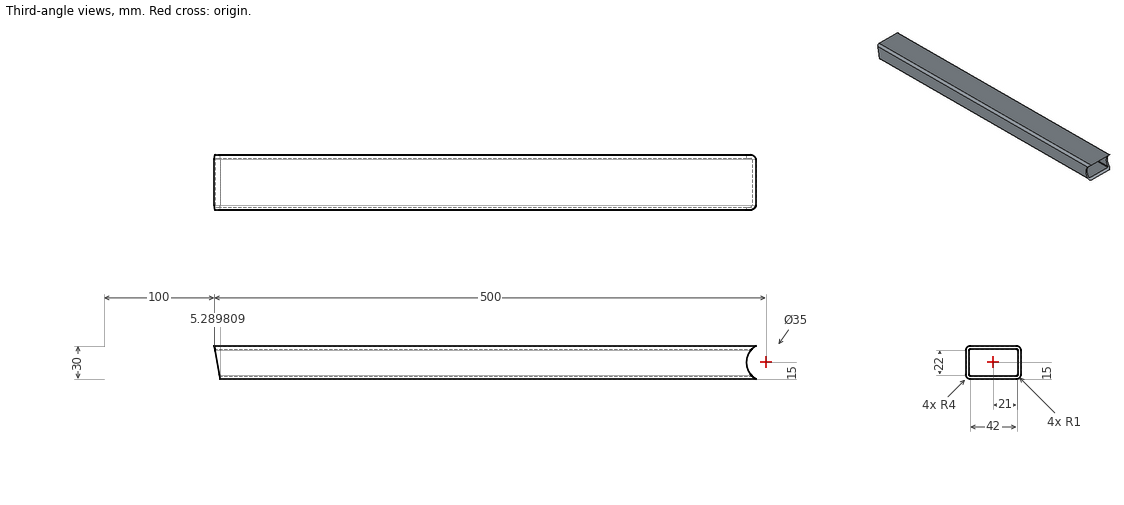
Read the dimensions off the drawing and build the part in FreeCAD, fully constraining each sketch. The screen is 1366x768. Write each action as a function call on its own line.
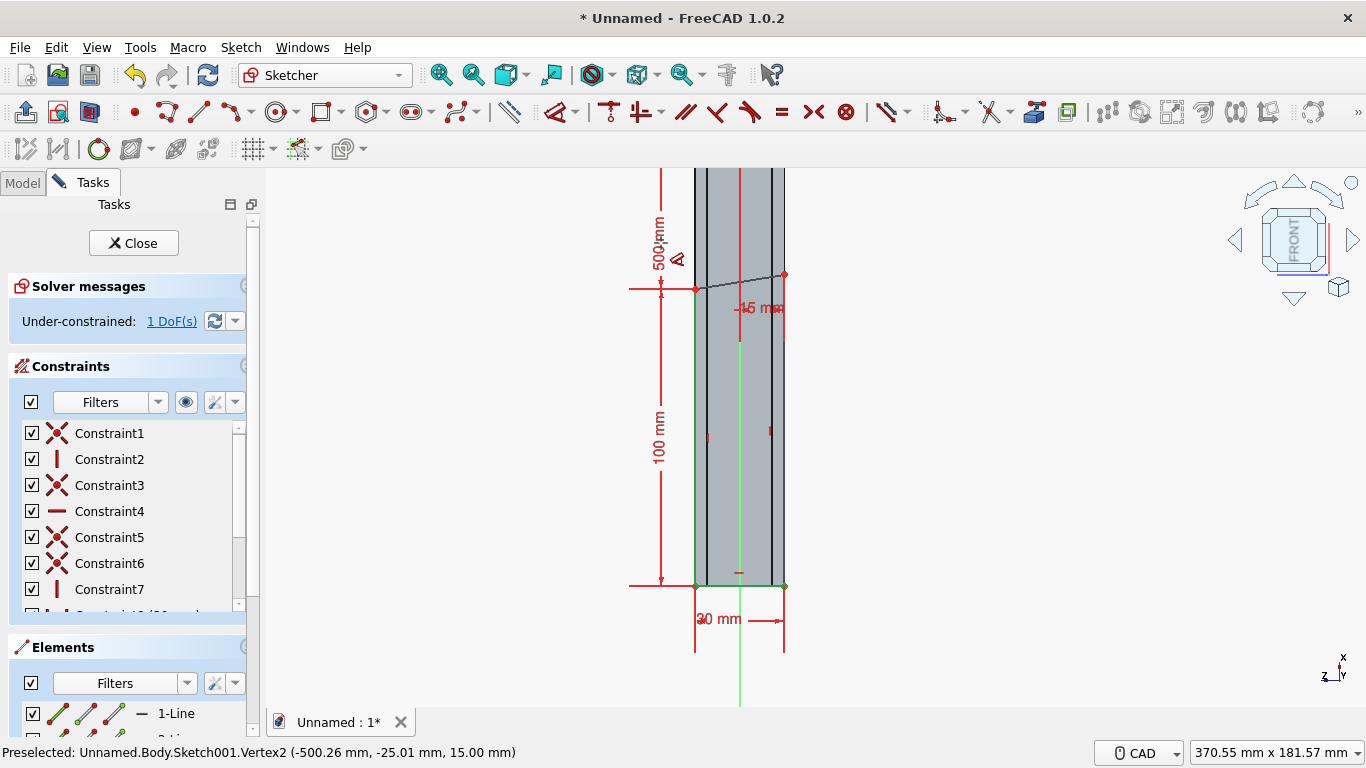
scroll(758, 279, up, 5)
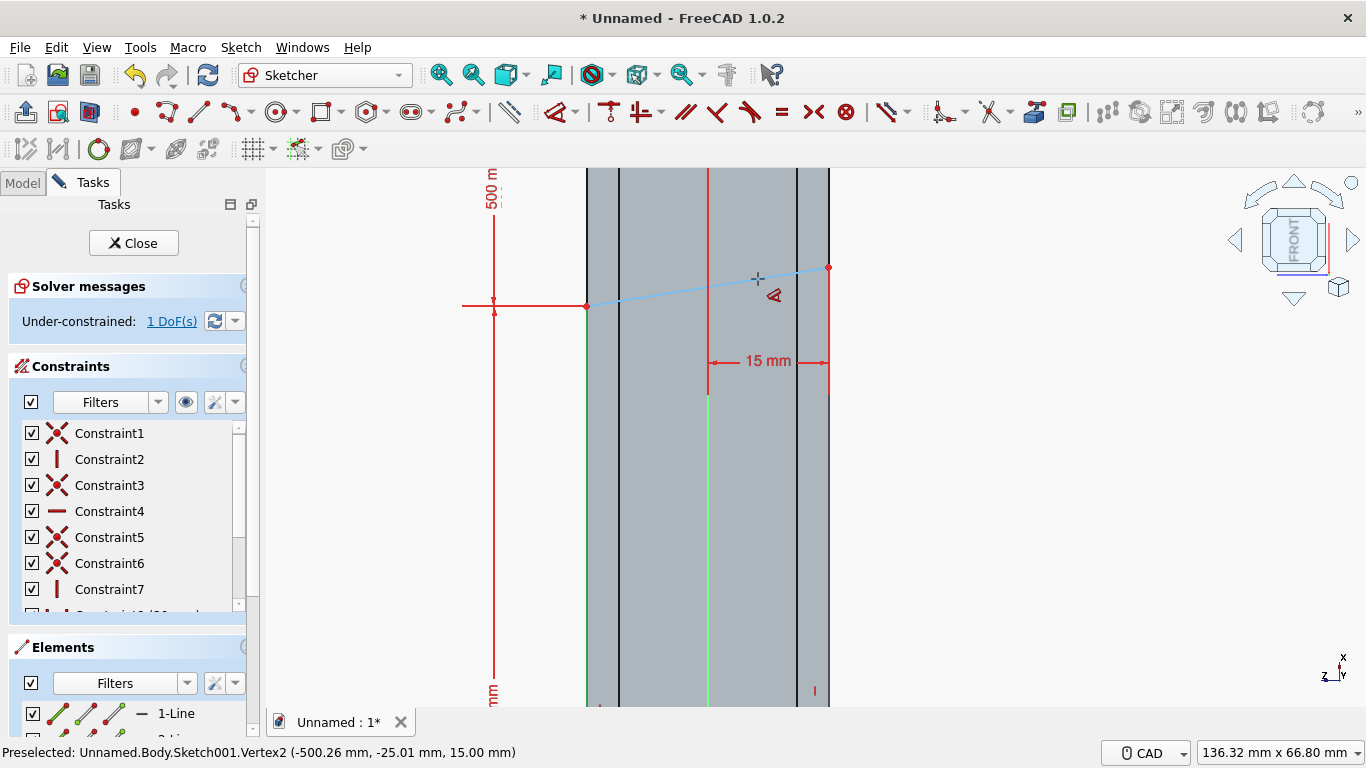
click(756, 279)
click(863, 287)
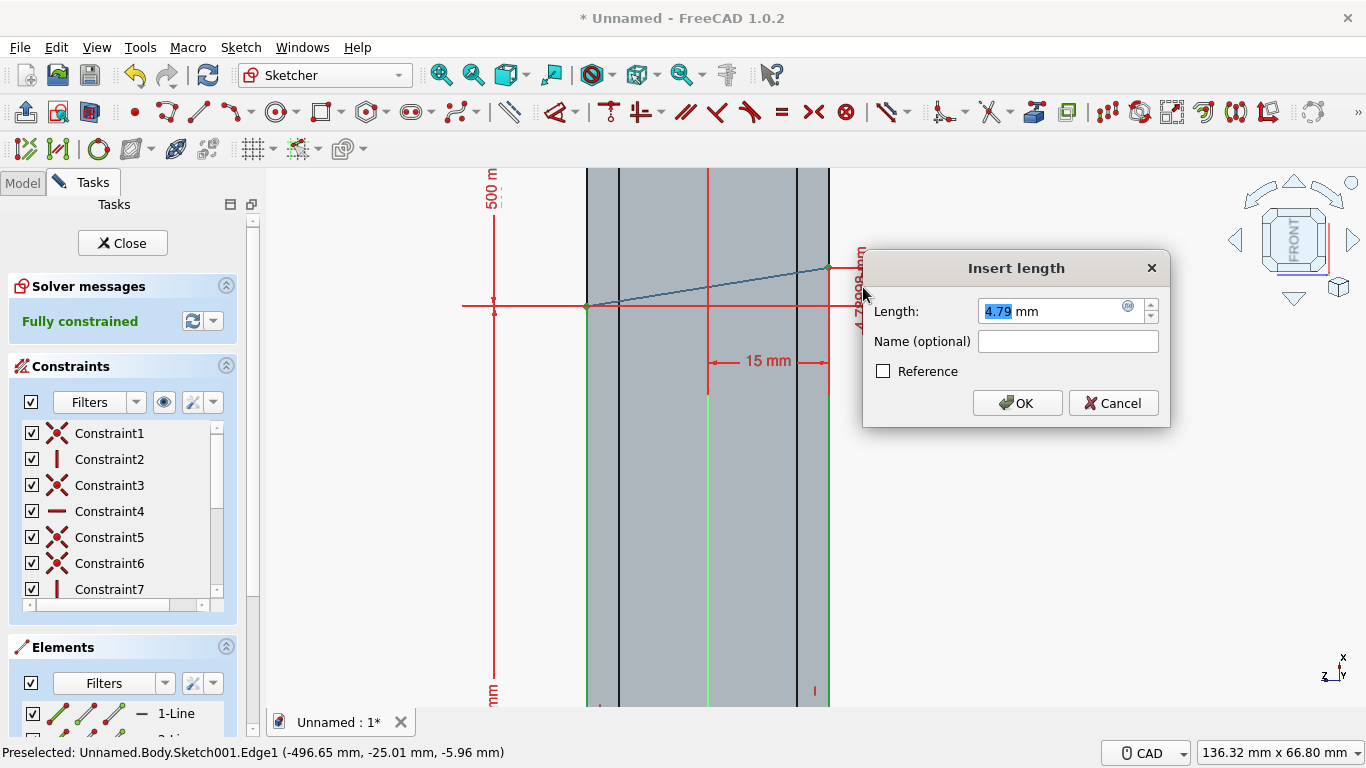
text(5.289809)
key(Return)
key(Escape)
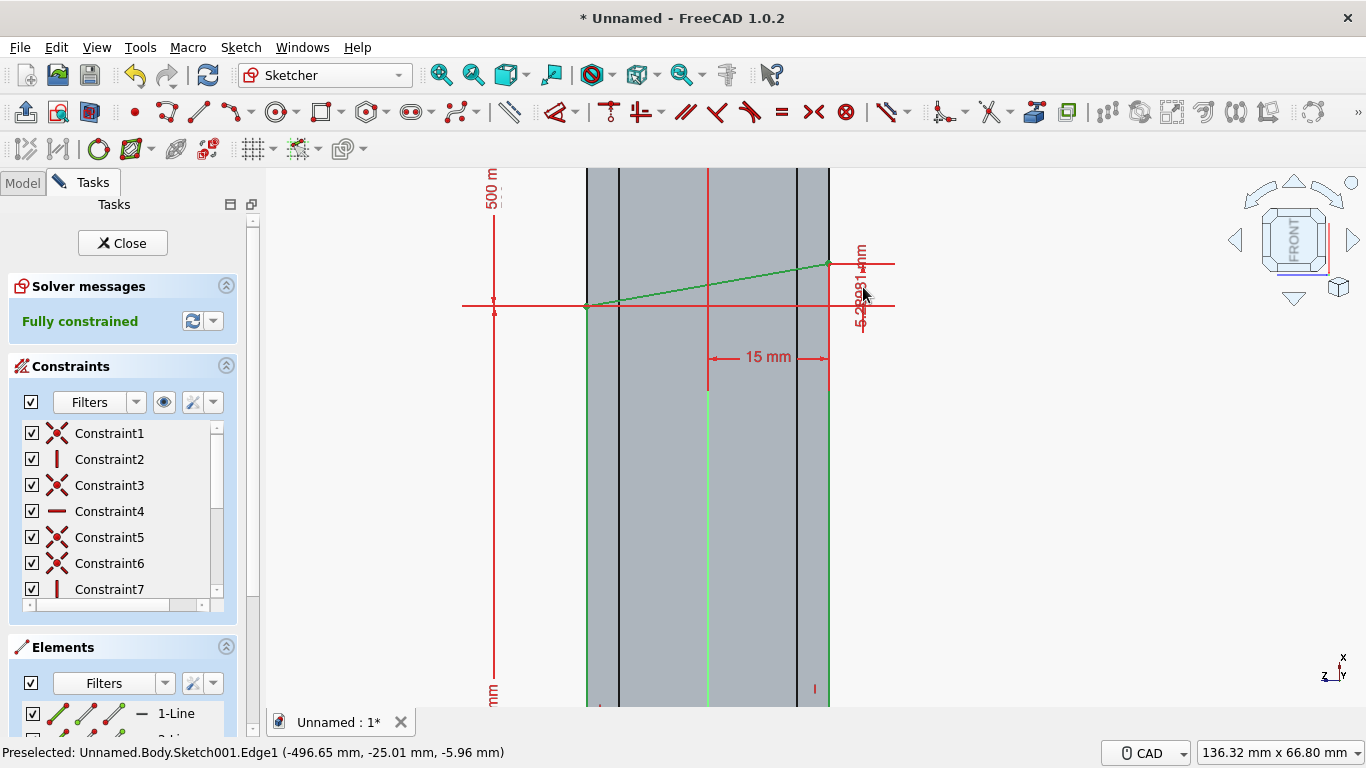
click(123, 243)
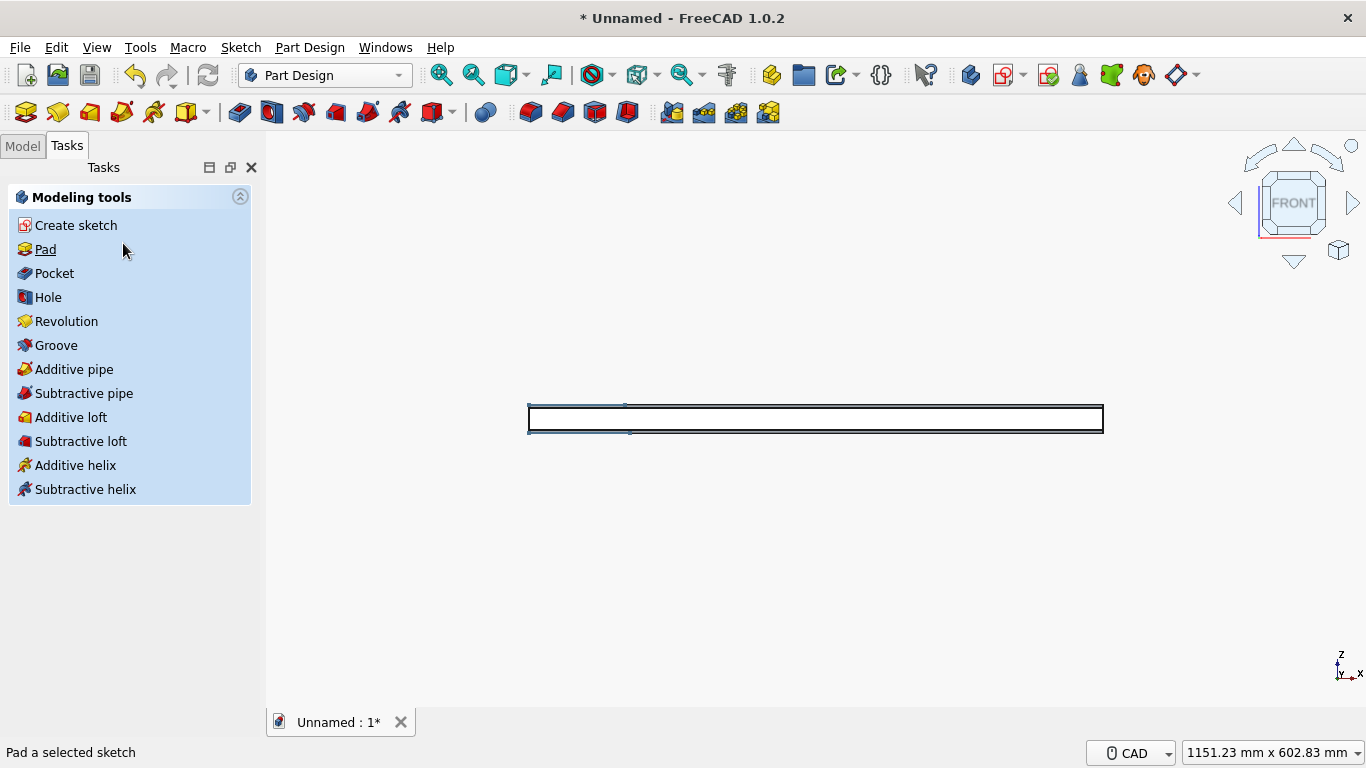
click(240, 112)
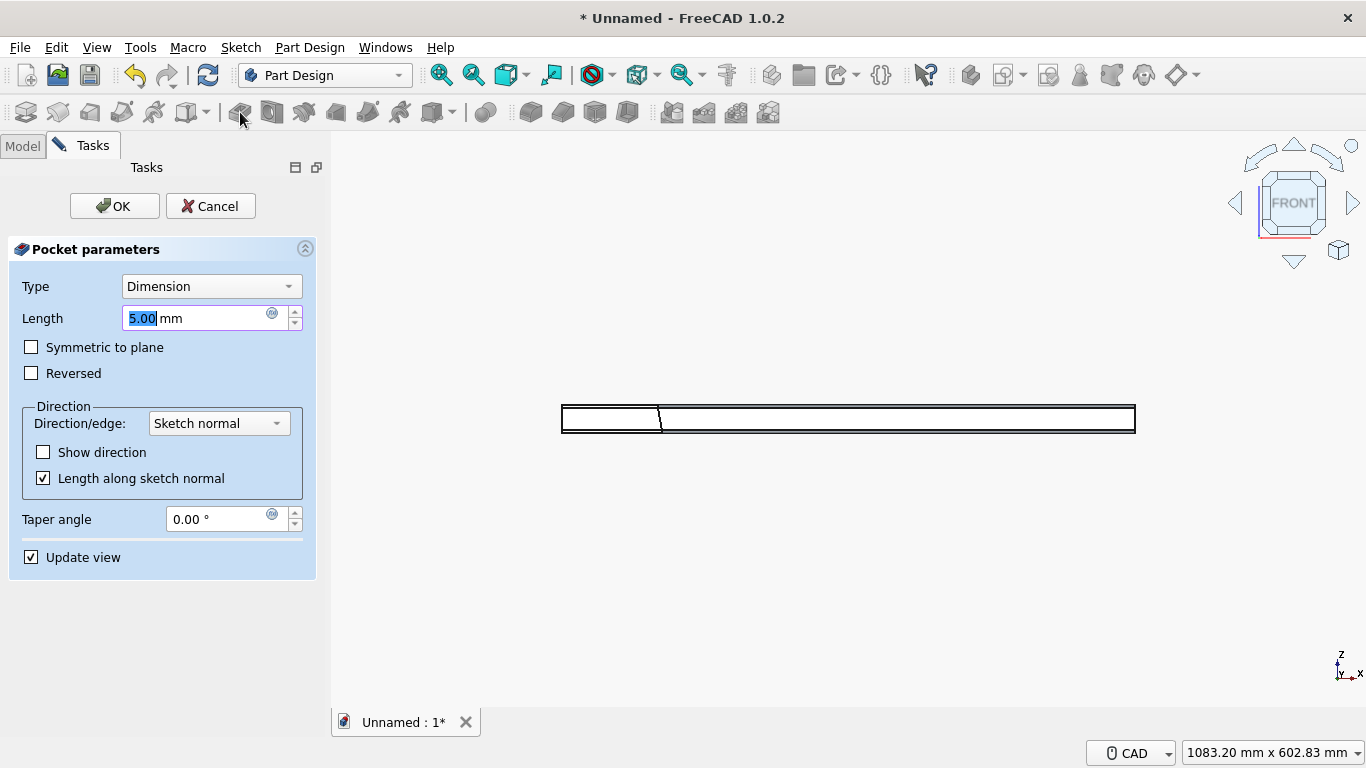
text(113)
key(Tab)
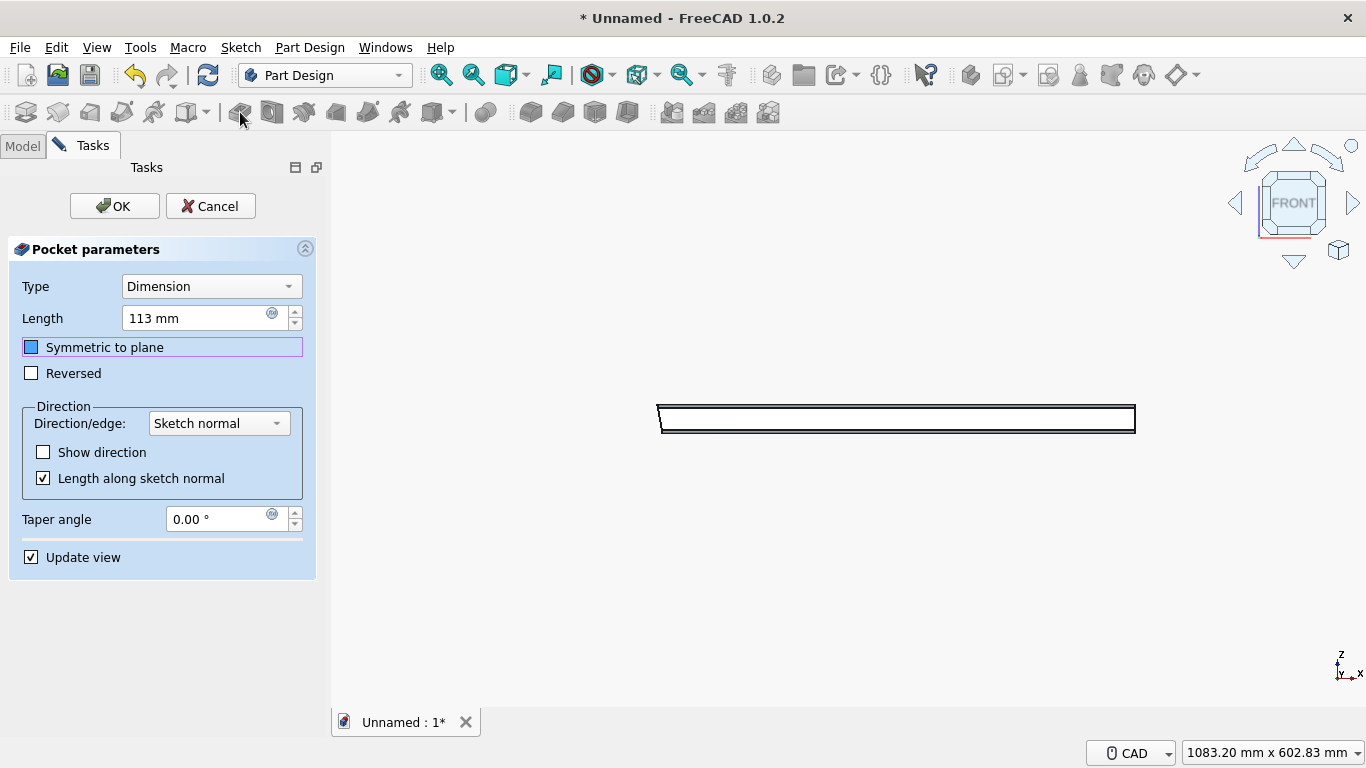
click(115, 206)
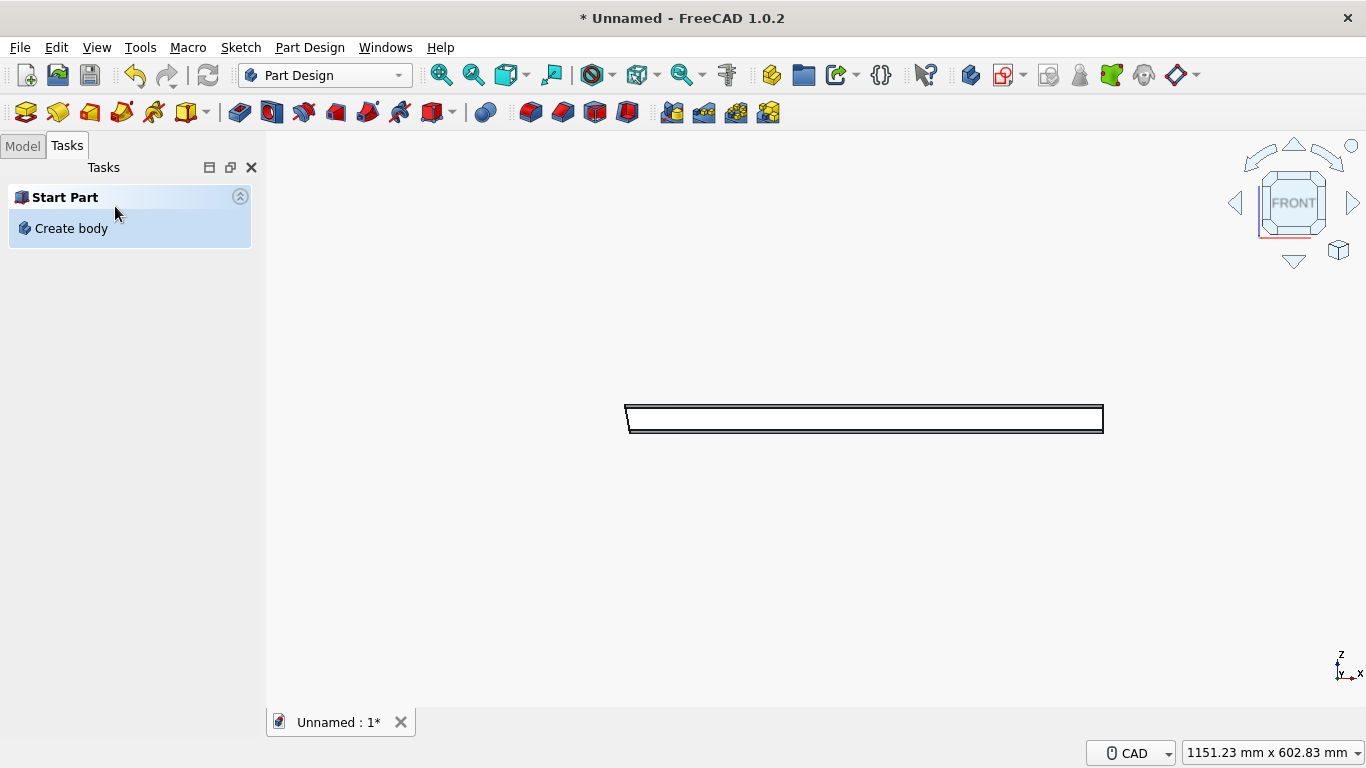
key(v)
key(f)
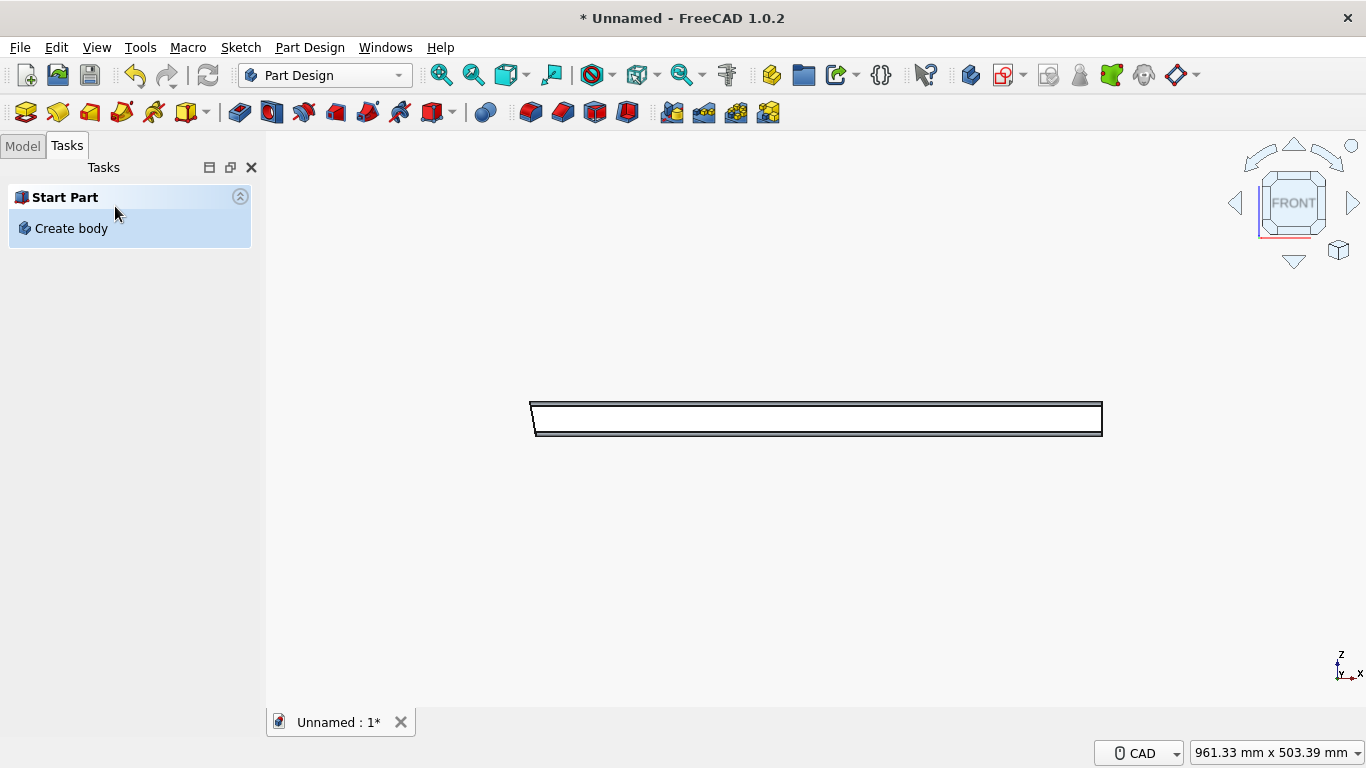
click(816, 418)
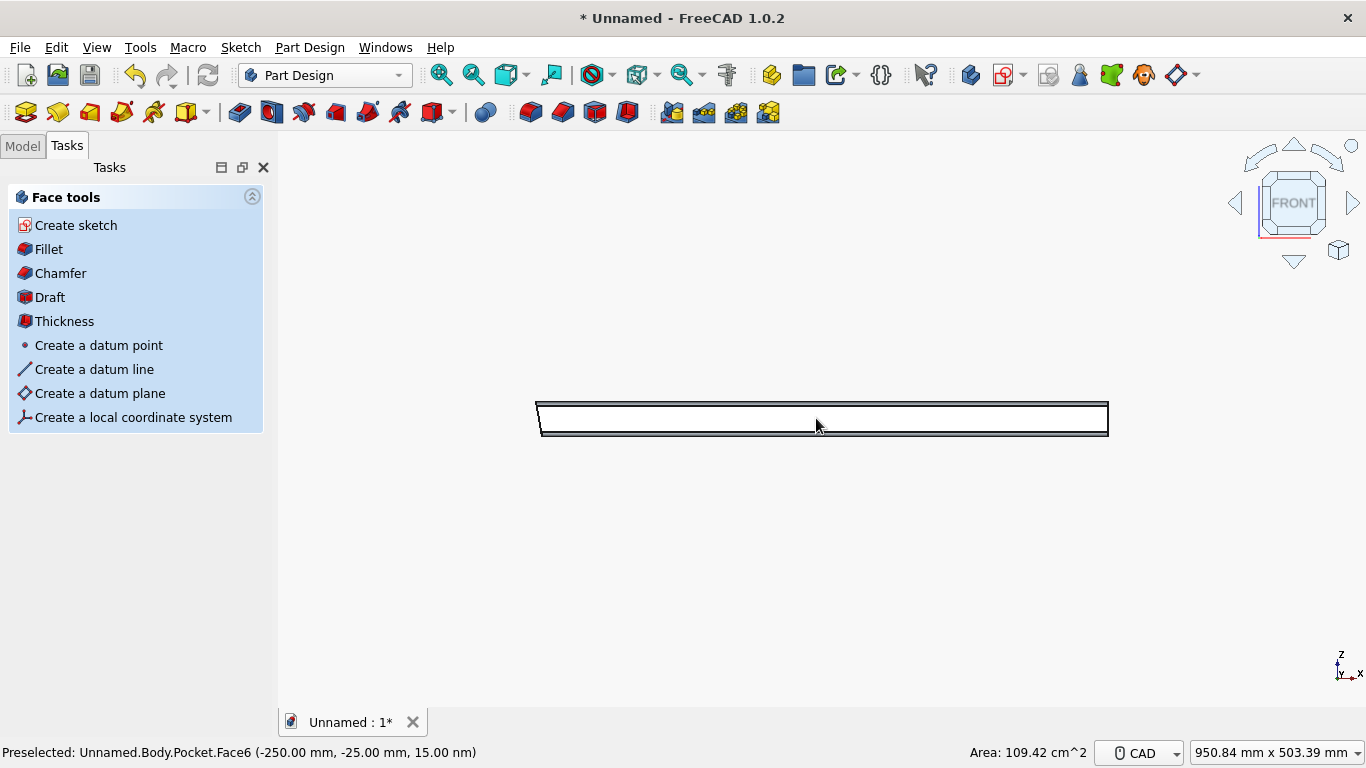
click(1004, 76)